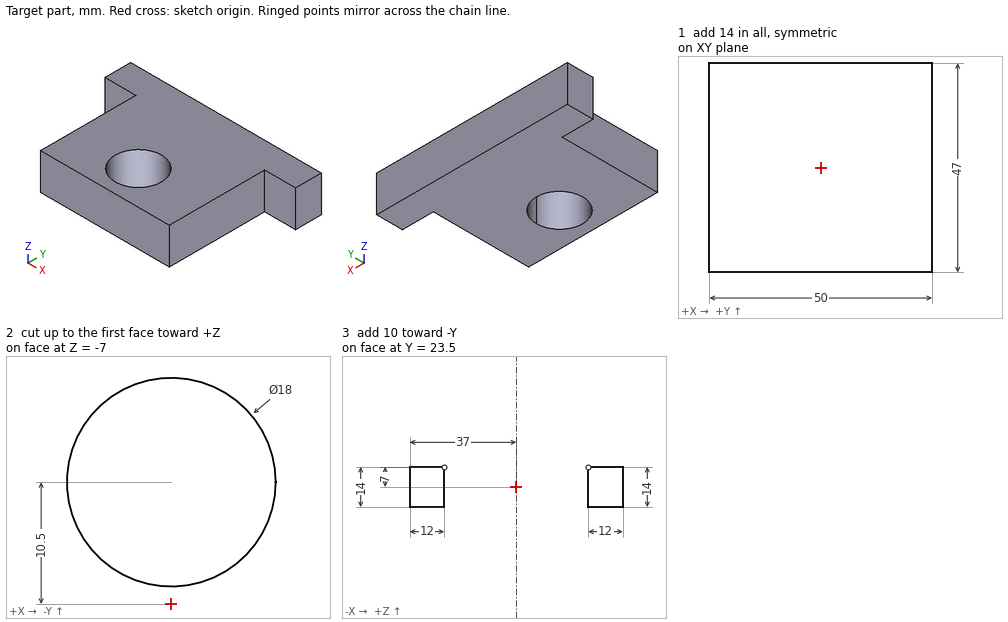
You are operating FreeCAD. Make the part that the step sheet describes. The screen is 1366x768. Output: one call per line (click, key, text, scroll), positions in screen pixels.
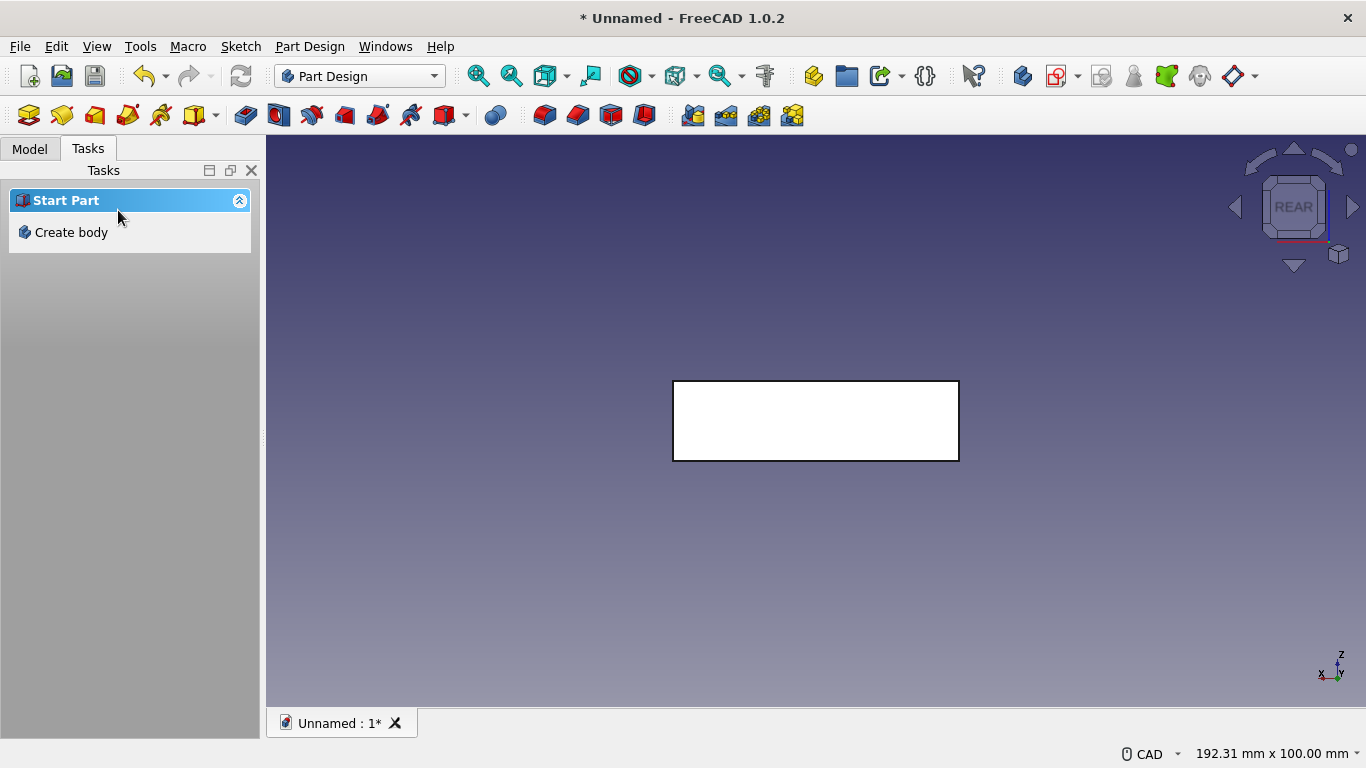
click(479, 76)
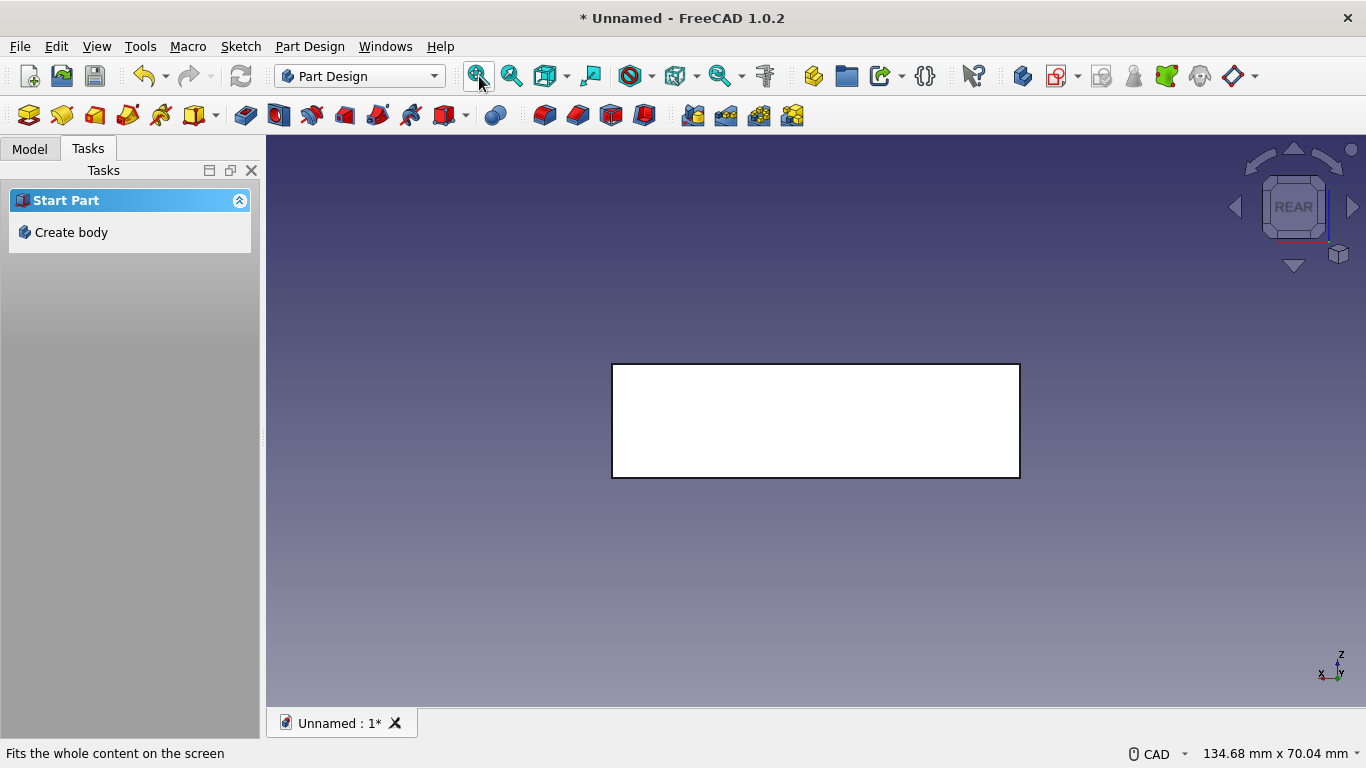
click(699, 420)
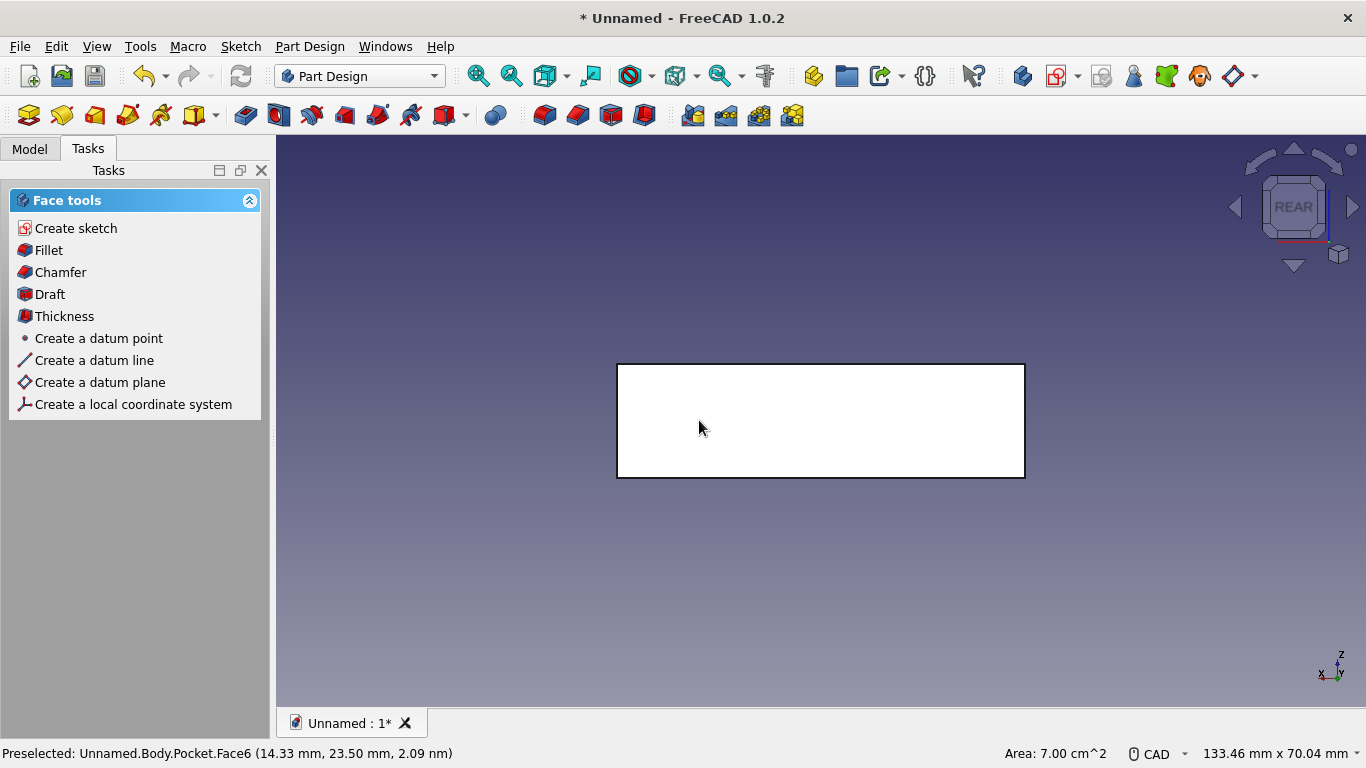
click(1056, 76)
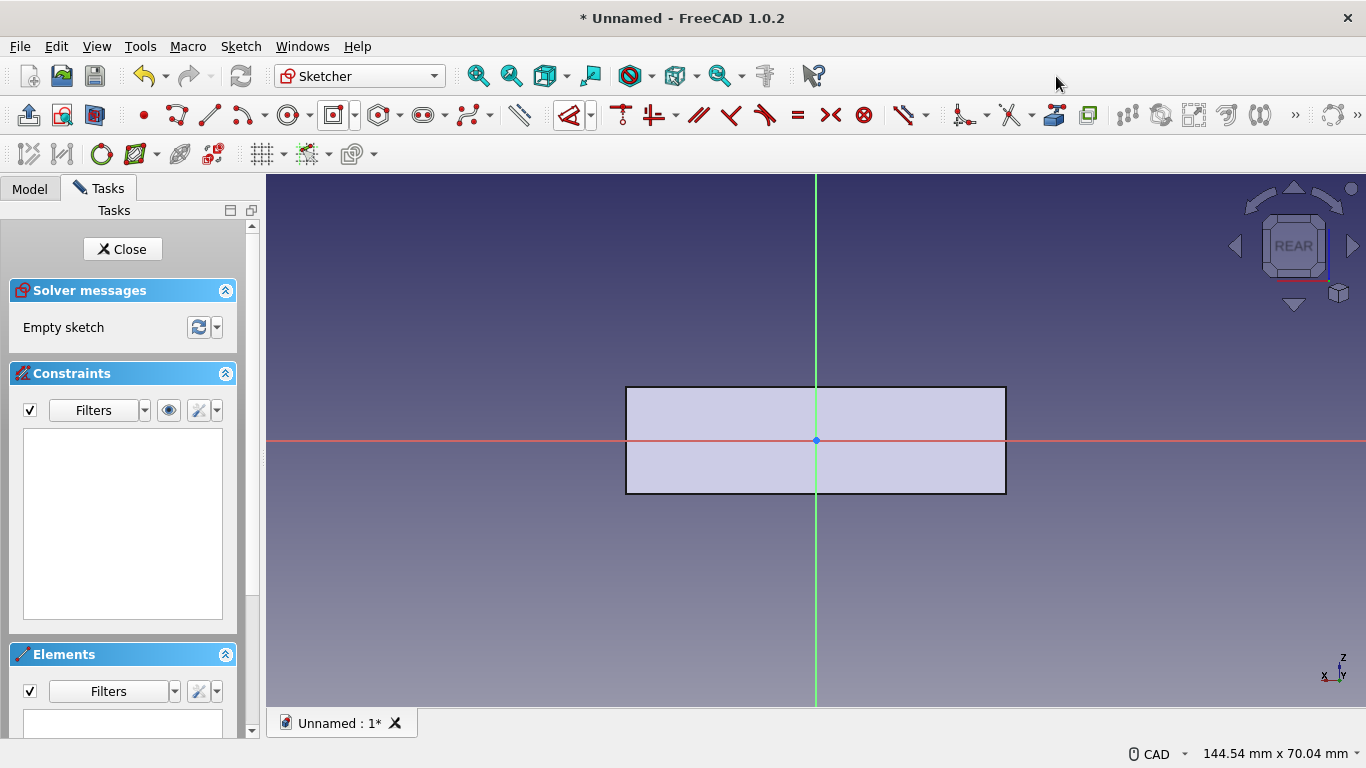
key(g)
key(r)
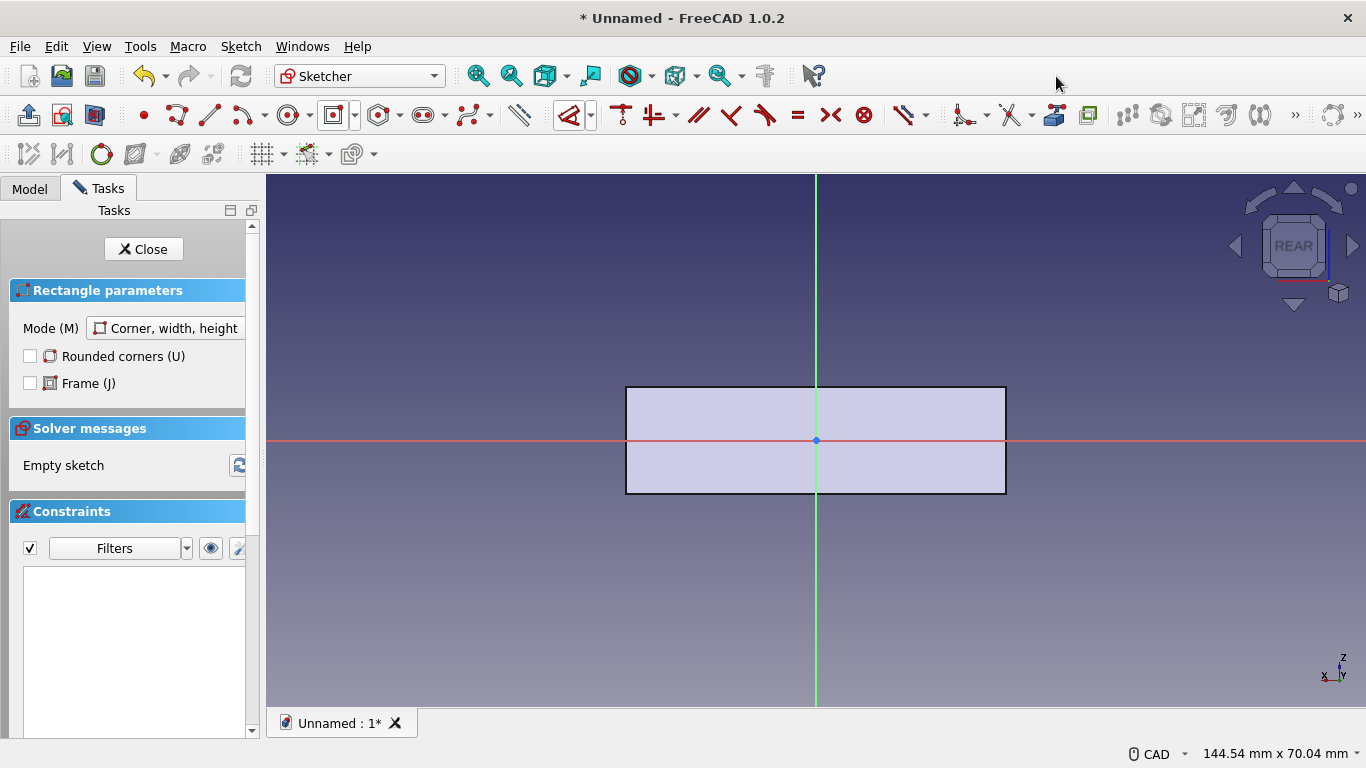
click(534, 387)
move(626, 494)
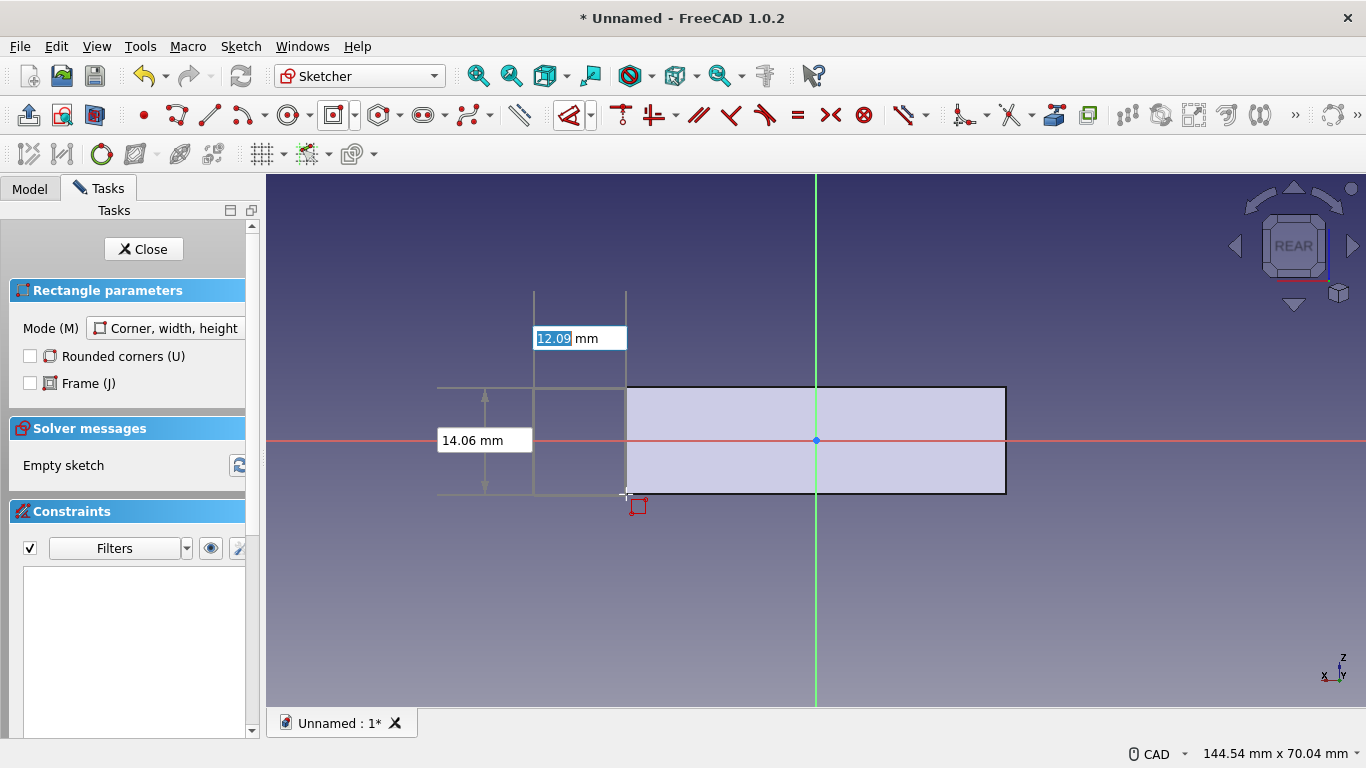
text(12)
key(Tab)
text(14)
key(Return)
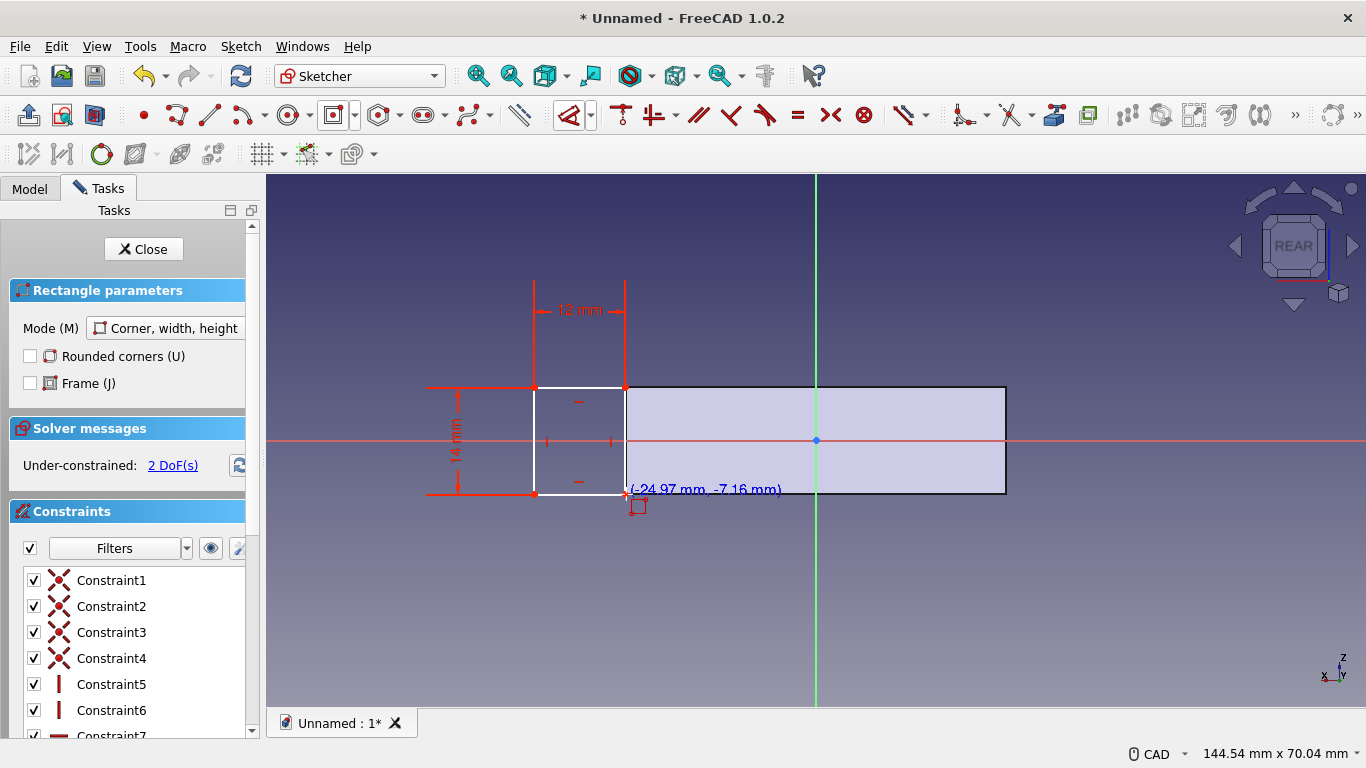
click(1006, 387)
move(1098, 494)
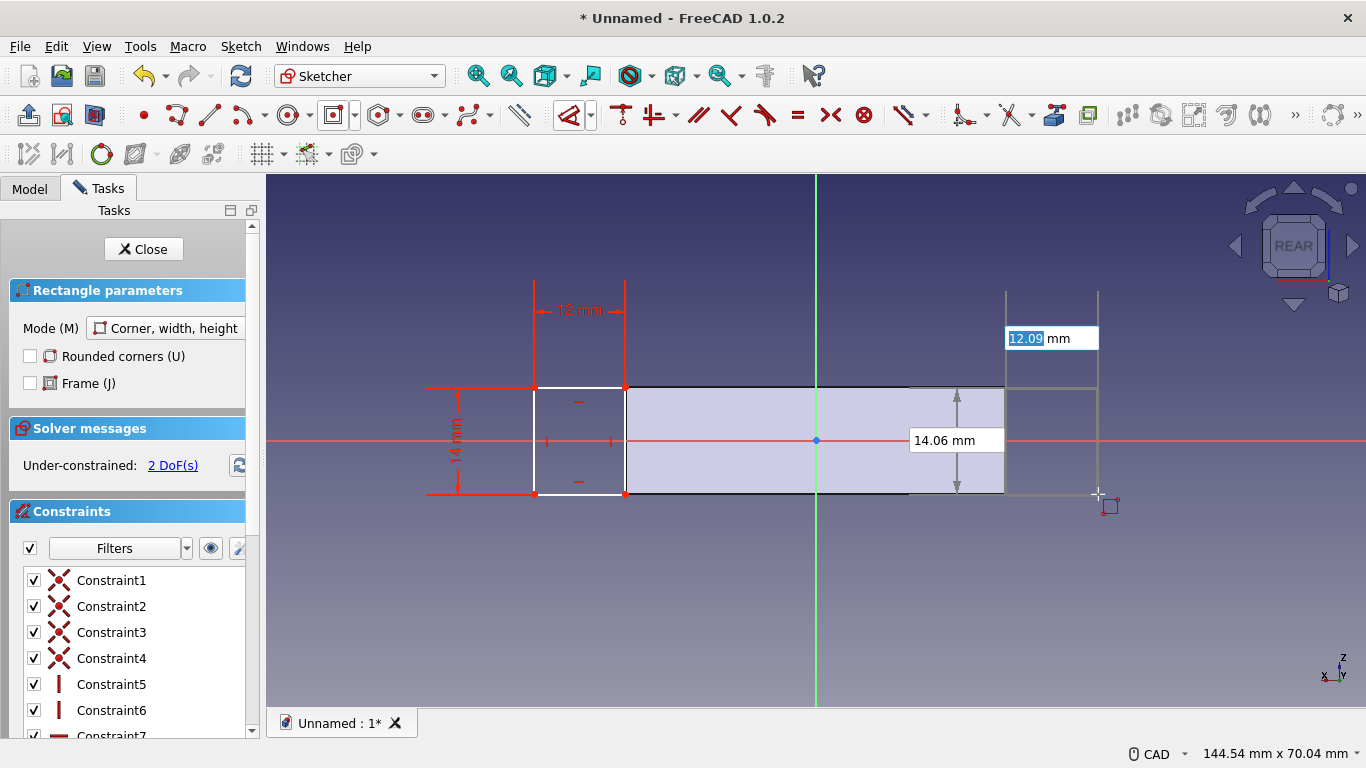
text(12)
key(Tab)
text(14)
key(Return)
key(Escape)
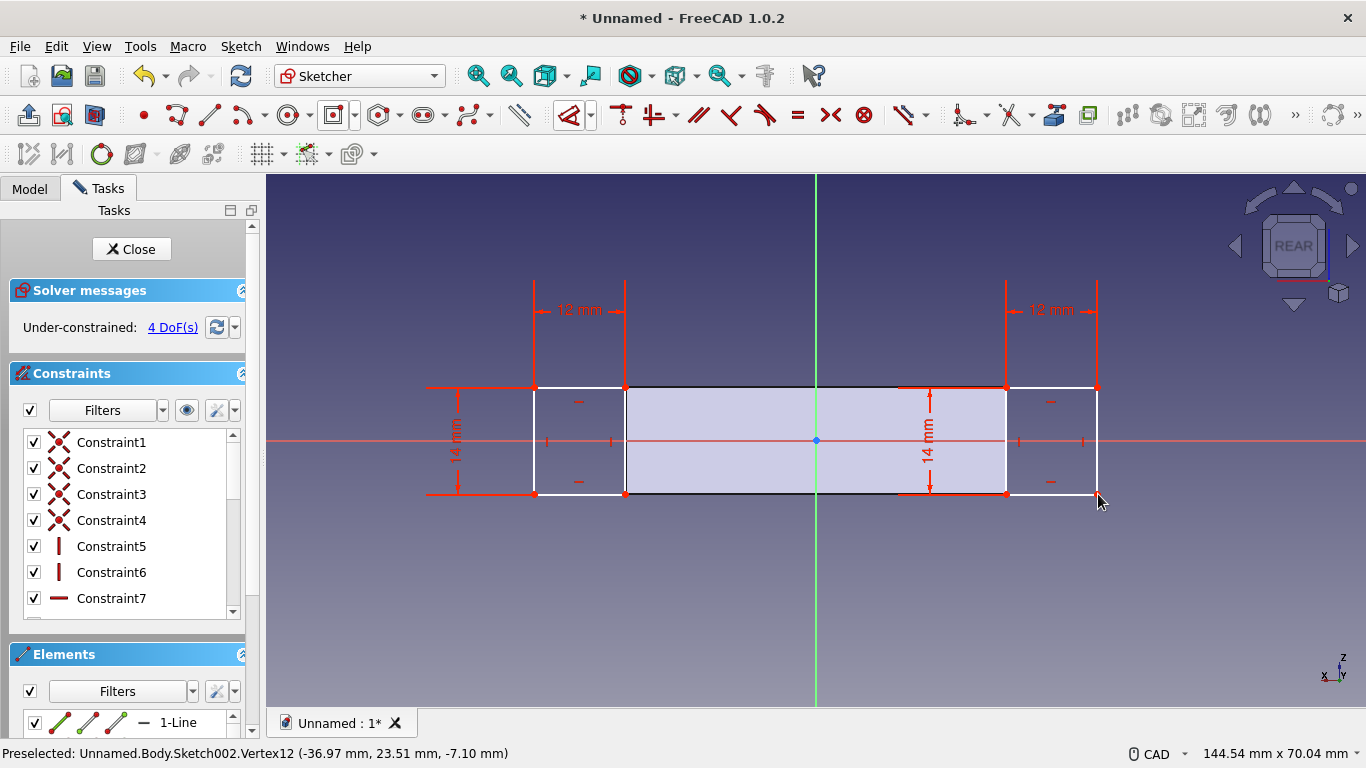
click(625, 388)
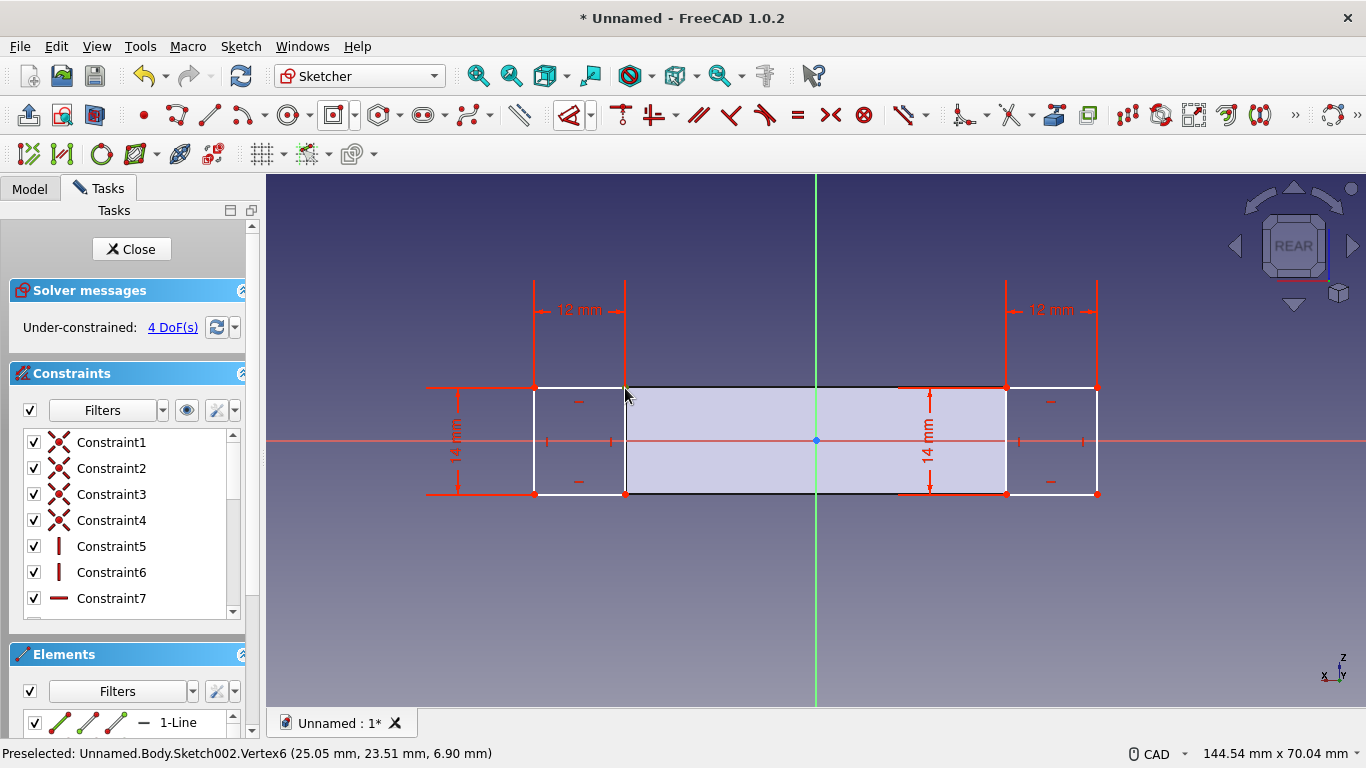
click(1006, 388)